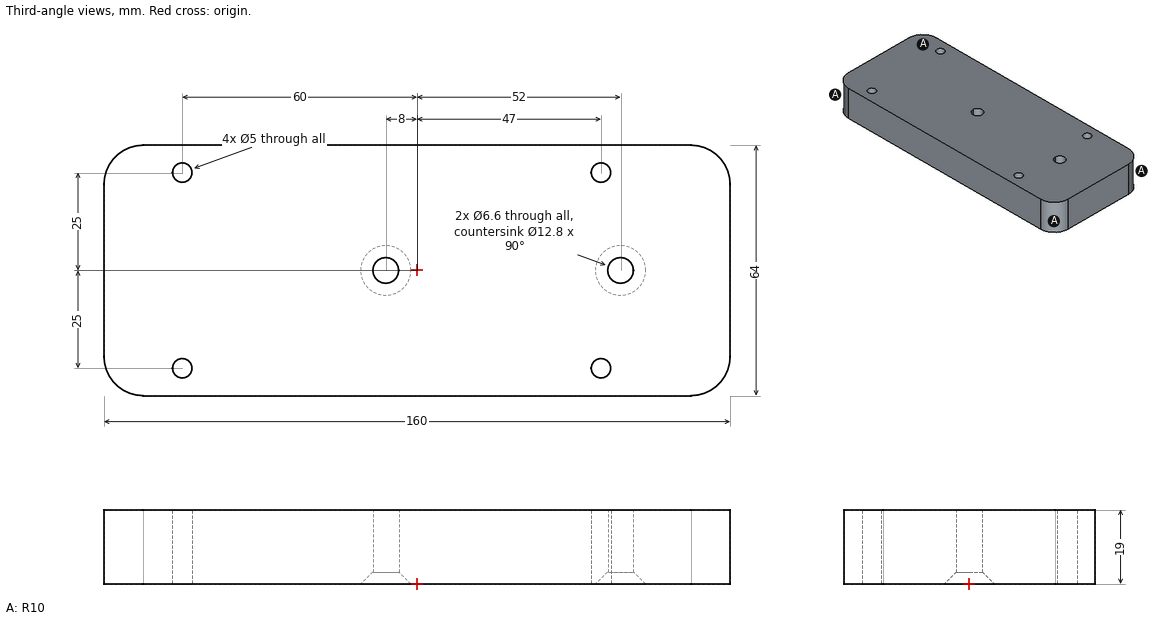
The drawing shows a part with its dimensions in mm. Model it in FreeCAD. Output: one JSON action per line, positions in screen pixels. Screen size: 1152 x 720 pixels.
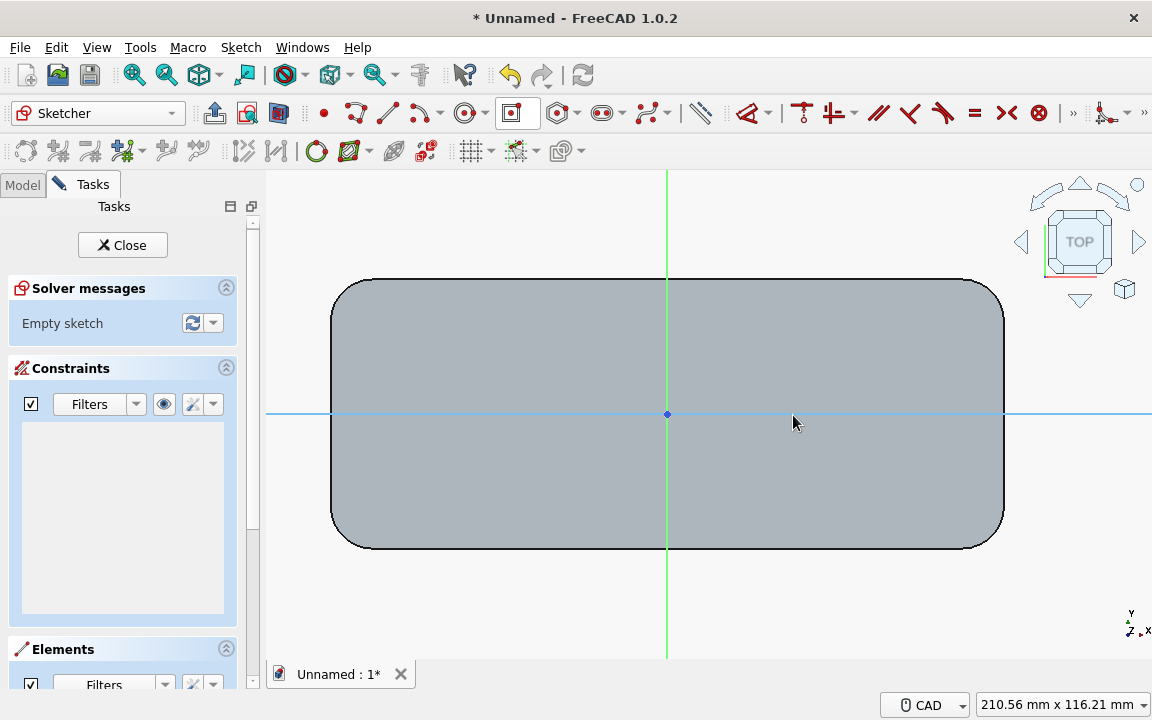
{"action": "key", "text": "g c"}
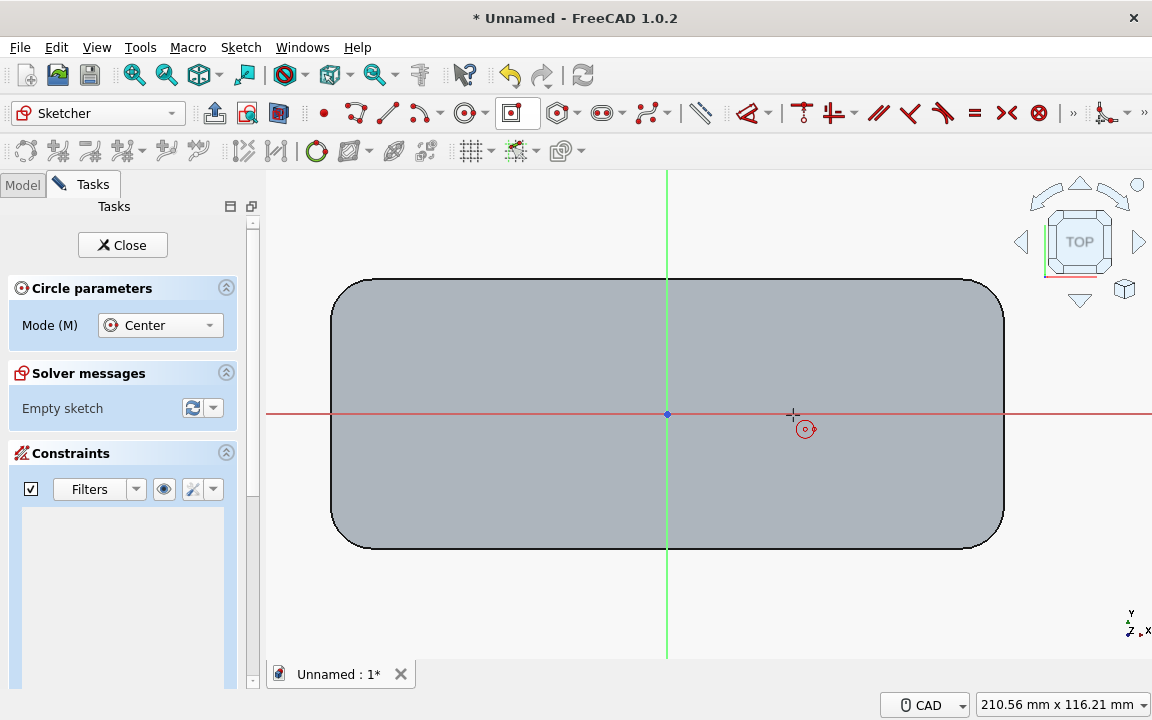
{"action": "scroll", "coordinate": [415, 309], "scroll_direction": "up", "scroll_amount": 4}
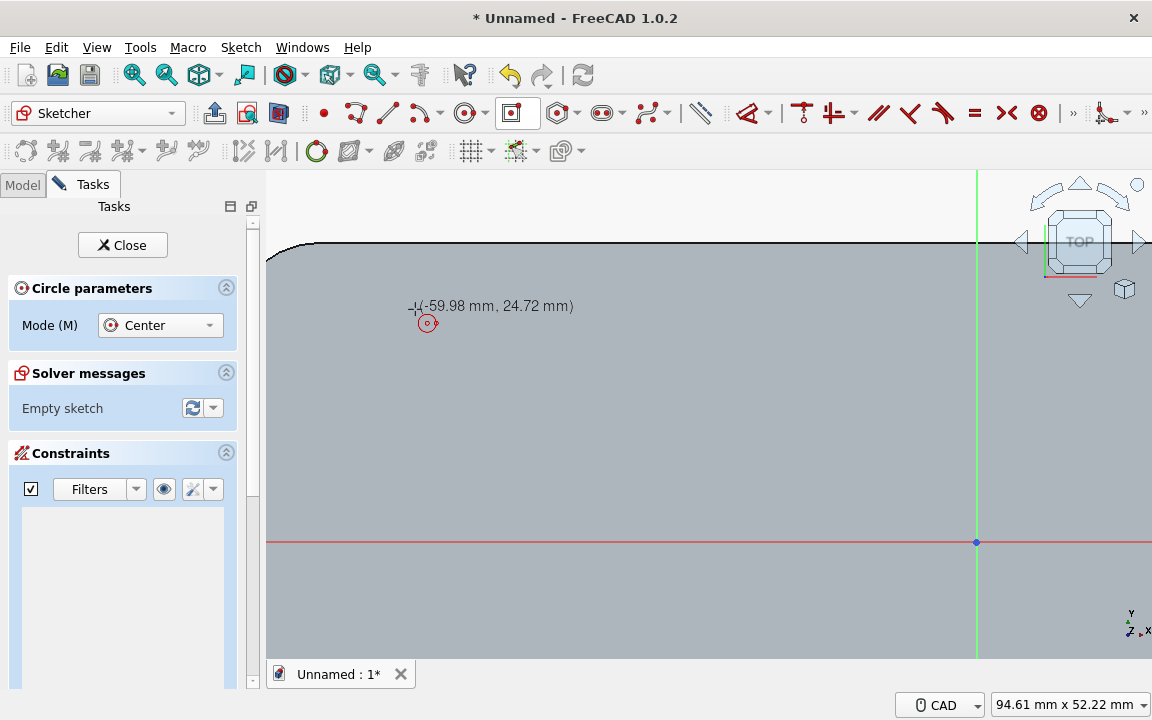
{"action": "left_click", "coordinate": [415, 308]}
{"action": "left_click", "coordinate": [431, 292]}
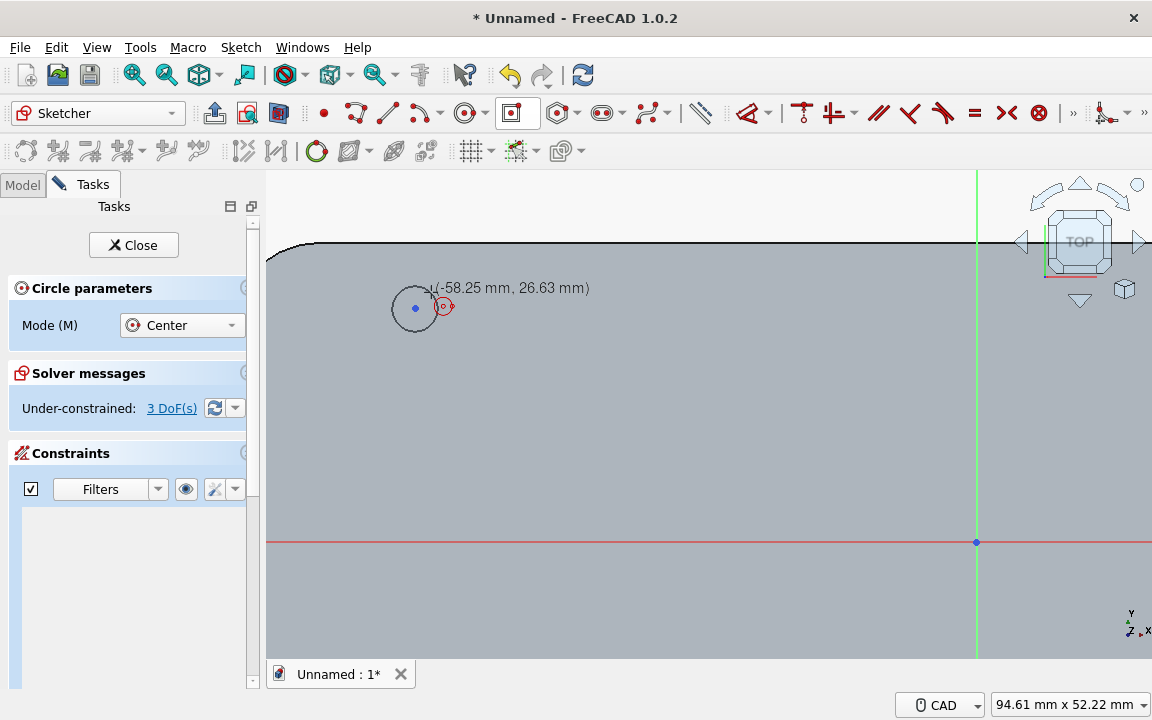
{"action": "scroll", "coordinate": [416, 310], "scroll_direction": "down", "scroll_amount": 4}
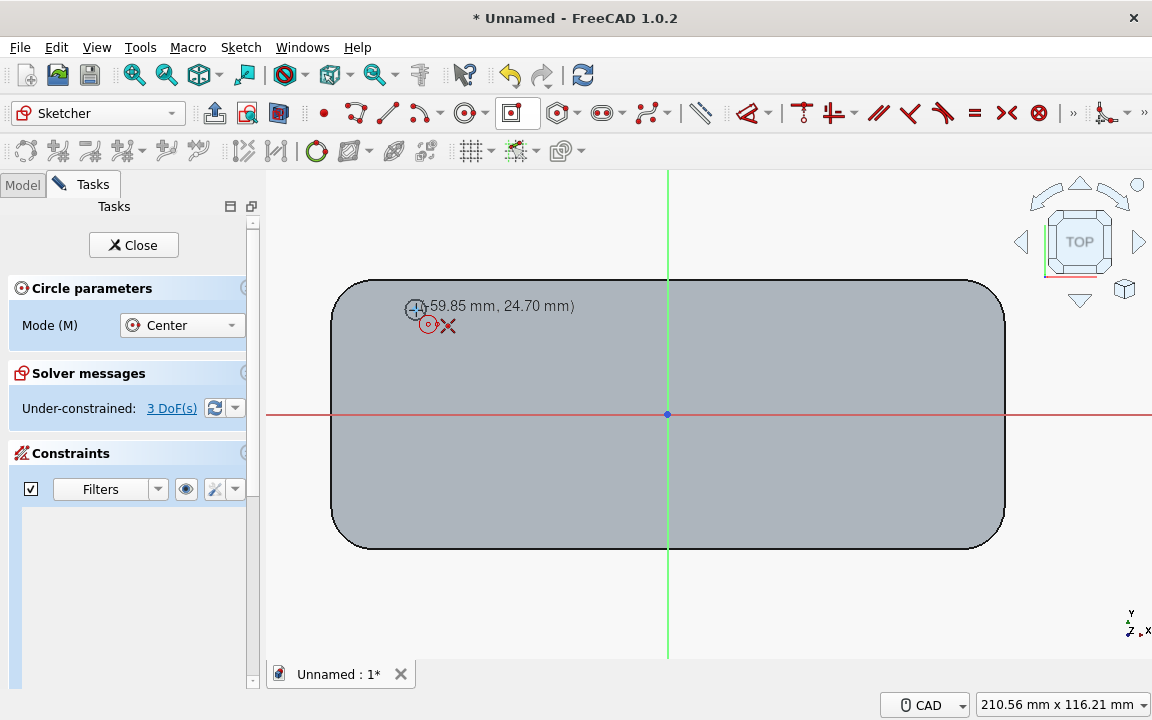
{"action": "scroll", "coordinate": [415, 520], "scroll_direction": "up", "scroll_amount": 4}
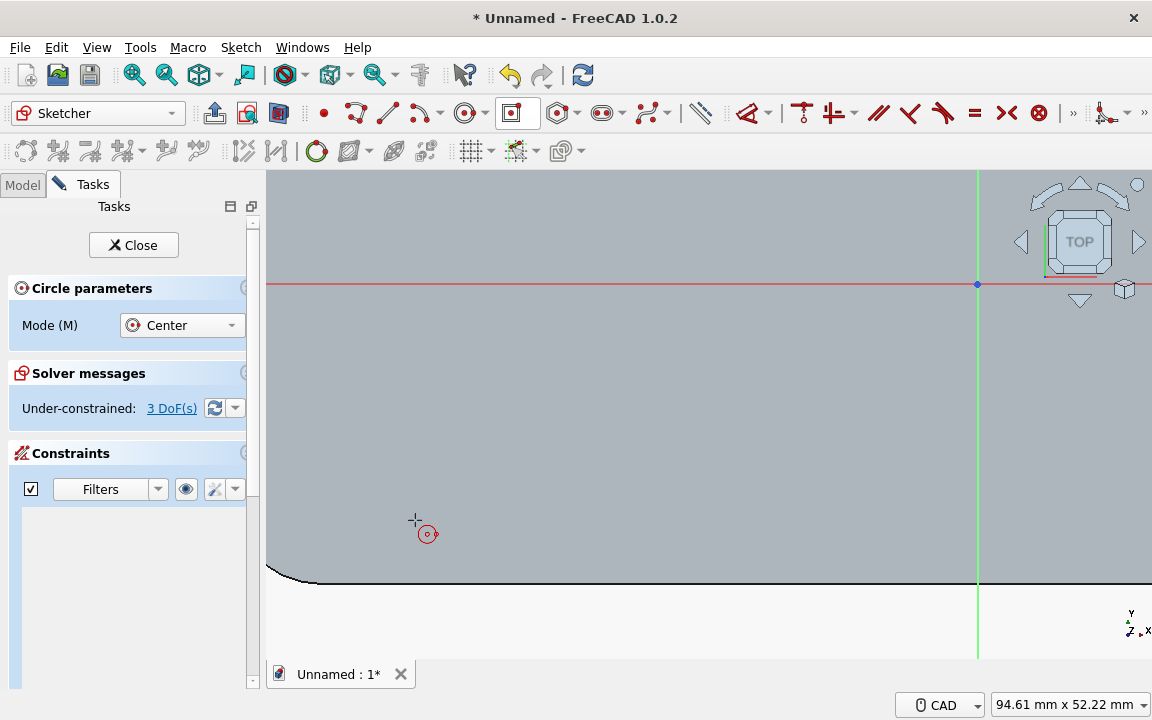
{"action": "left_click", "coordinate": [416, 519]}
{"action": "left_click", "coordinate": [432, 502]}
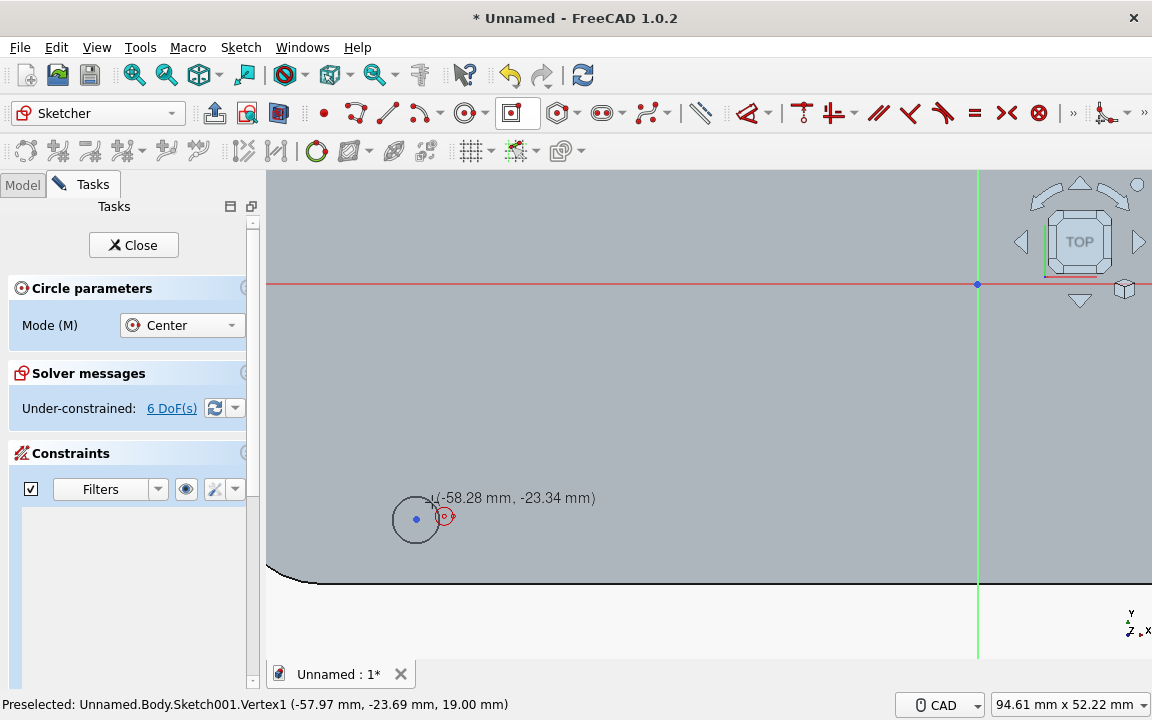
{"action": "scroll", "coordinate": [415, 521], "scroll_direction": "down", "scroll_amount": 4}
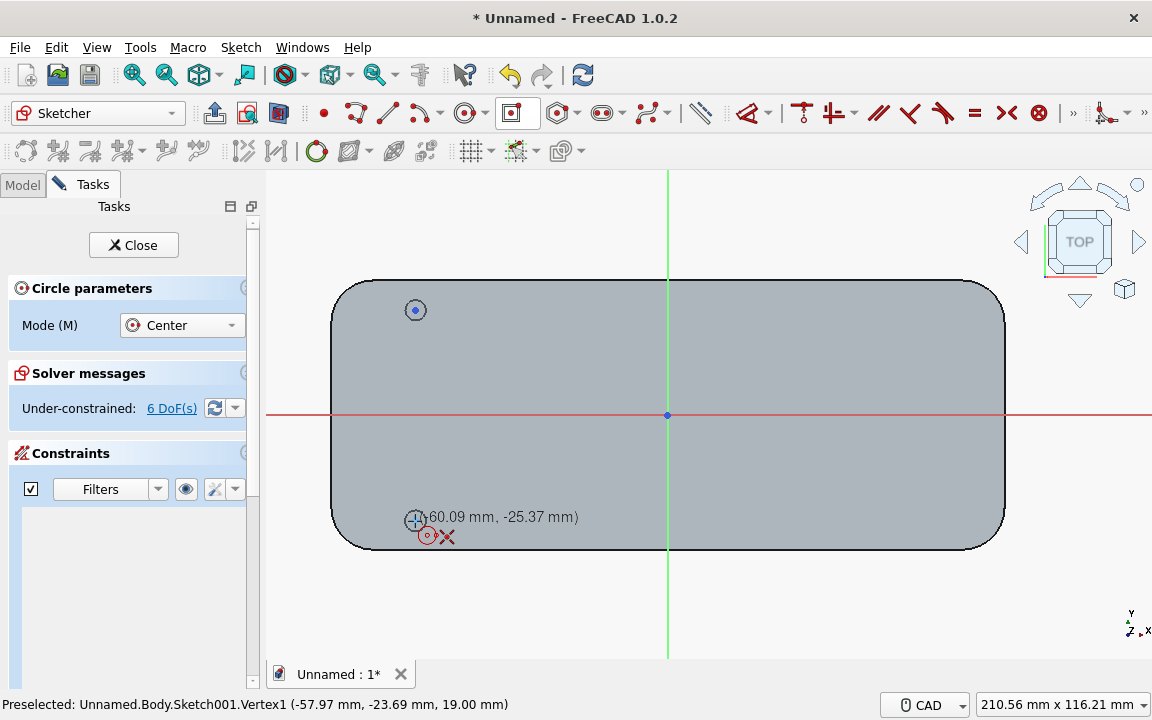
{"action": "scroll", "coordinate": [866, 310], "scroll_direction": "up", "scroll_amount": 4}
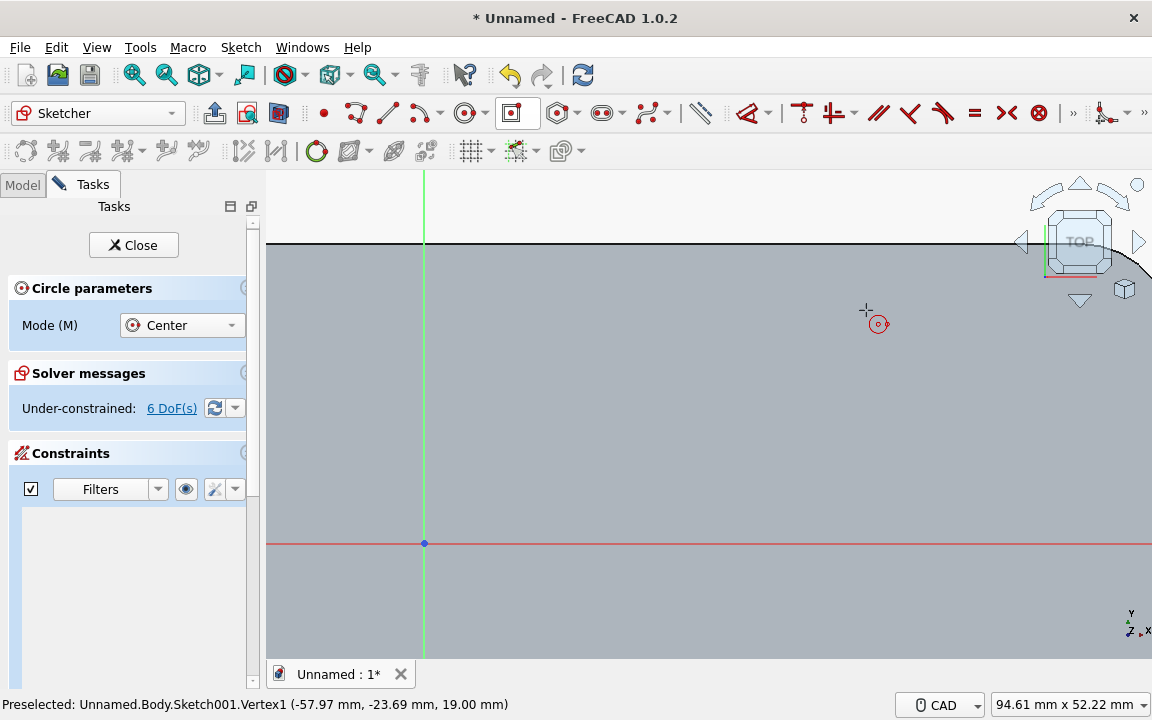
{"action": "left_click", "coordinate": [865, 309]}
{"action": "left_click", "coordinate": [881, 293]}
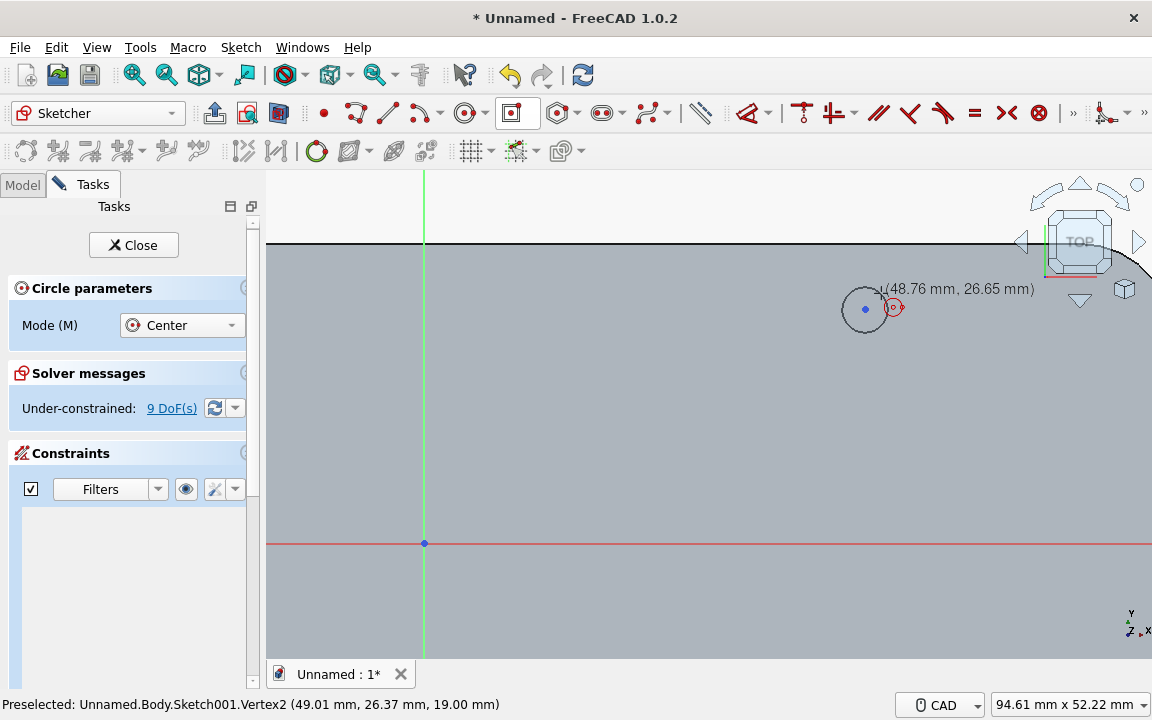
{"action": "scroll", "coordinate": [867, 309], "scroll_direction": "down", "scroll_amount": 4}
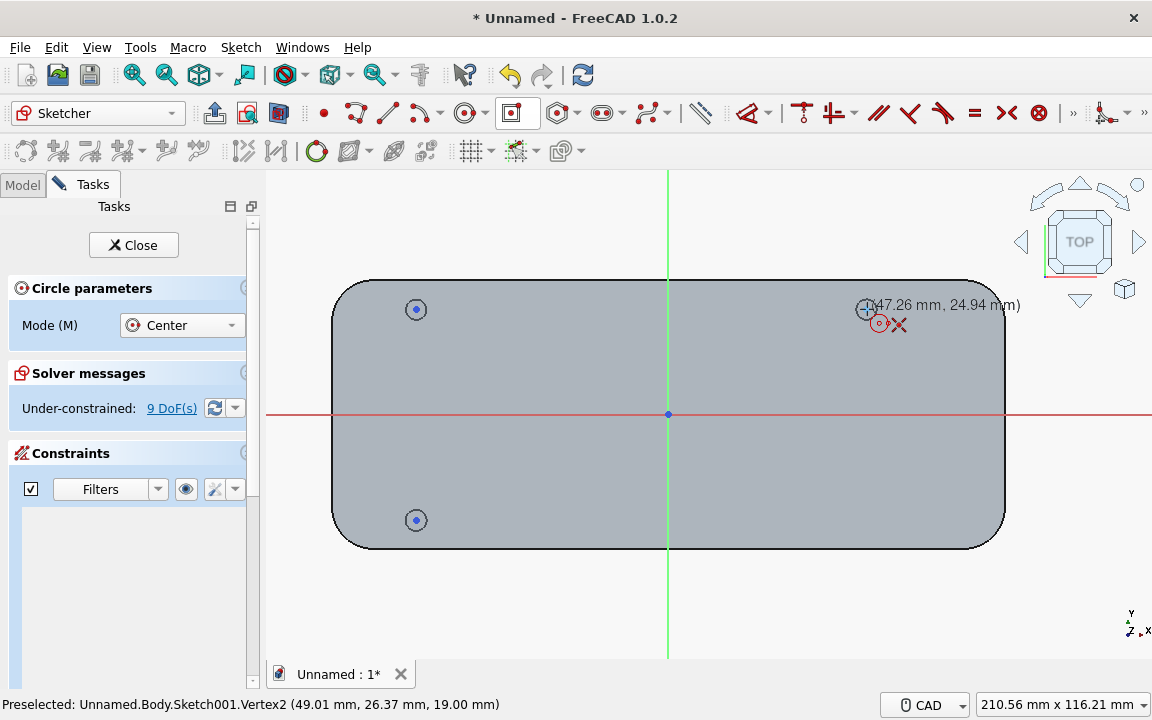
{"action": "scroll", "coordinate": [866, 520], "scroll_direction": "up", "scroll_amount": 4}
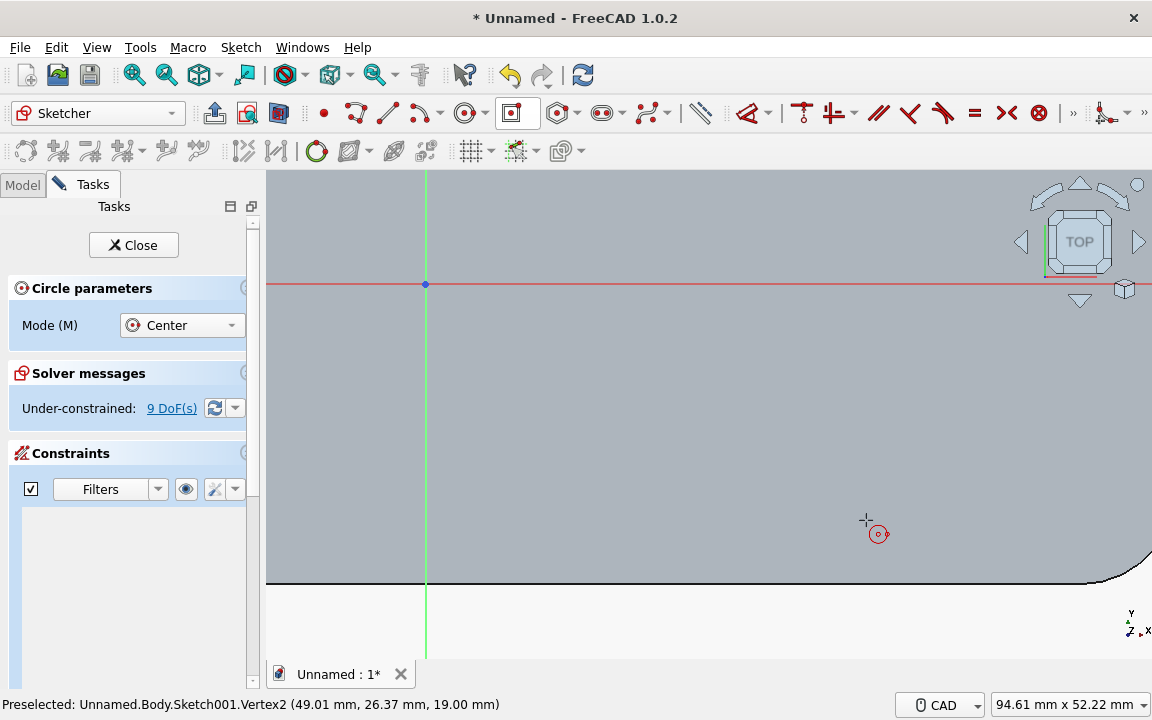
{"action": "left_click", "coordinate": [866, 519]}
{"action": "left_click", "coordinate": [882, 502]}
{"action": "key", "text": "Escape"}